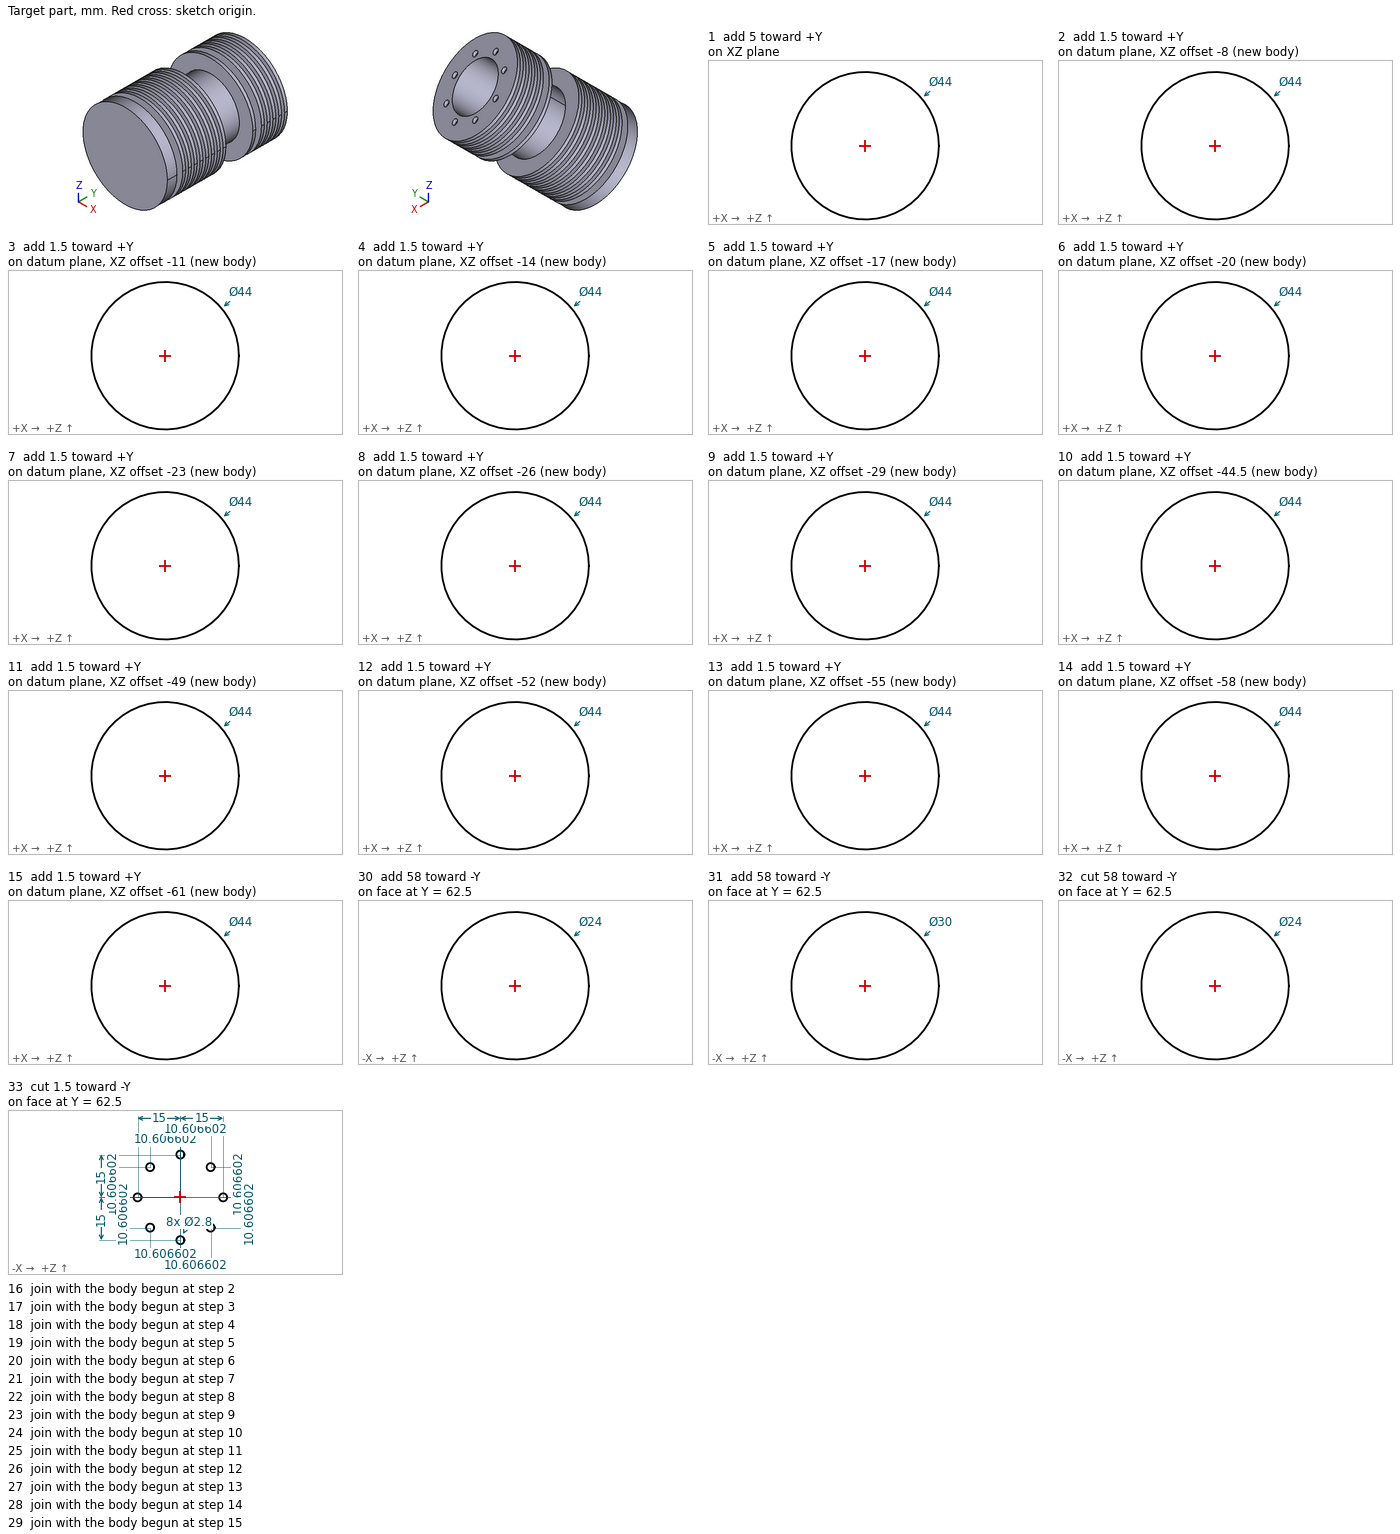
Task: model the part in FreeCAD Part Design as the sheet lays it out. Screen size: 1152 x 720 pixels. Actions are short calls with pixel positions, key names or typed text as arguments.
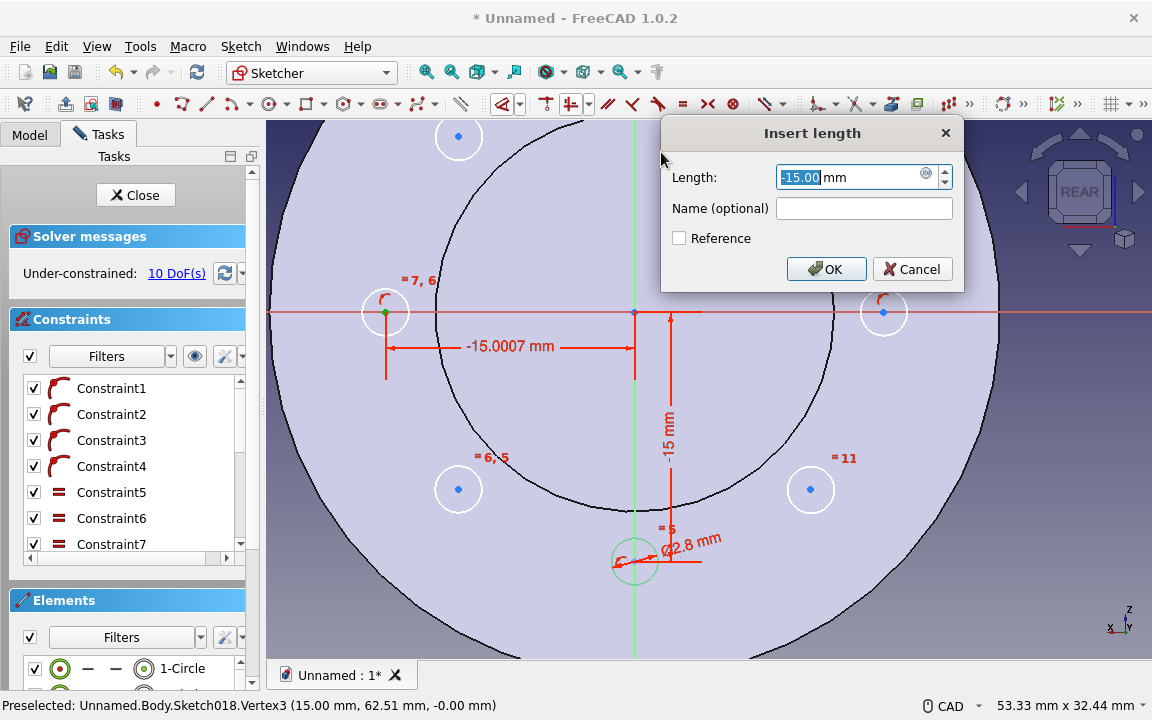
text(-15)
key(Return)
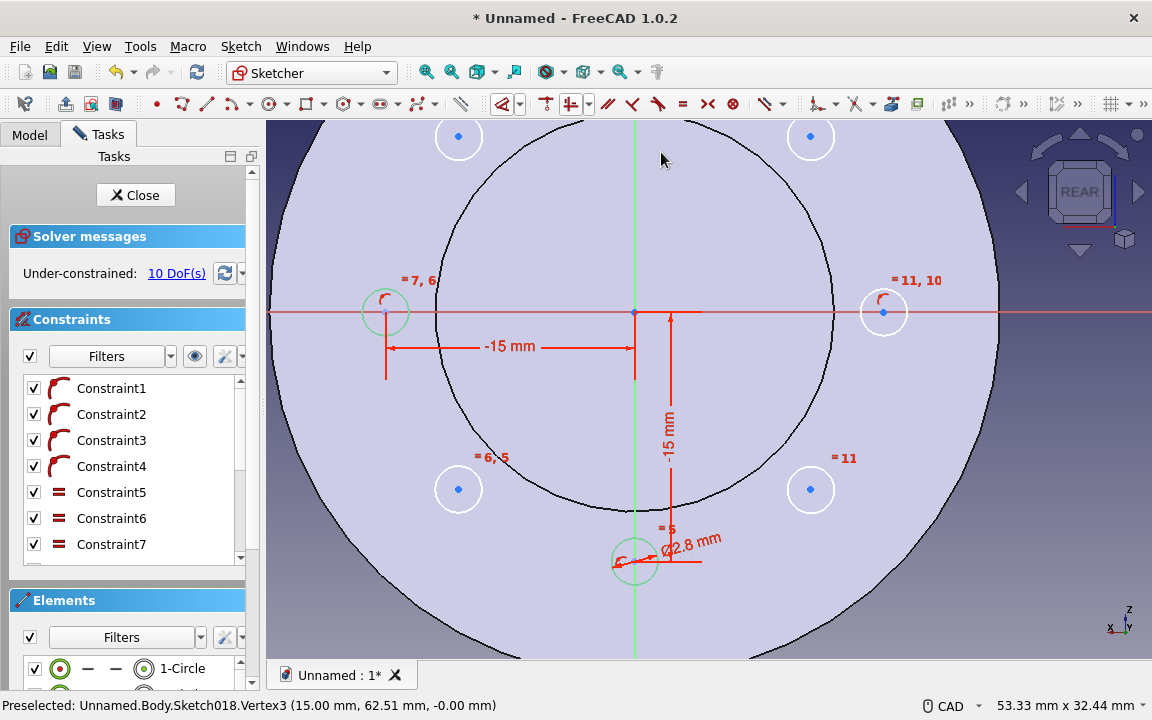
scroll(652, 546, down, 2)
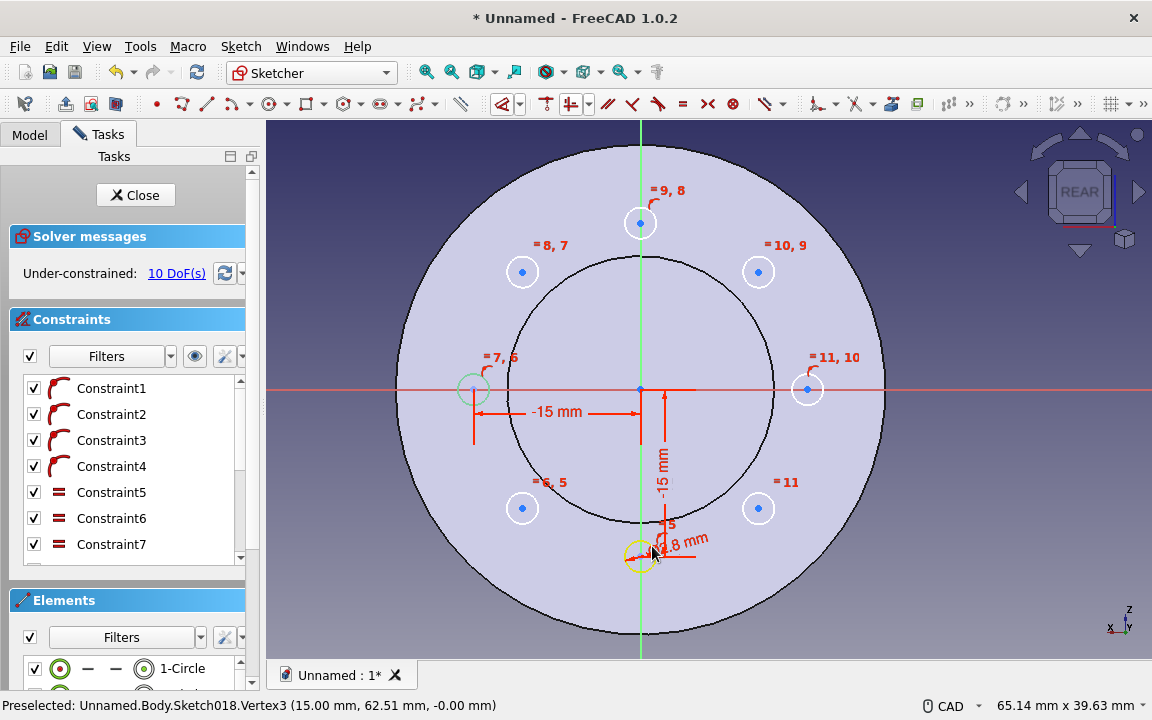
click(641, 223)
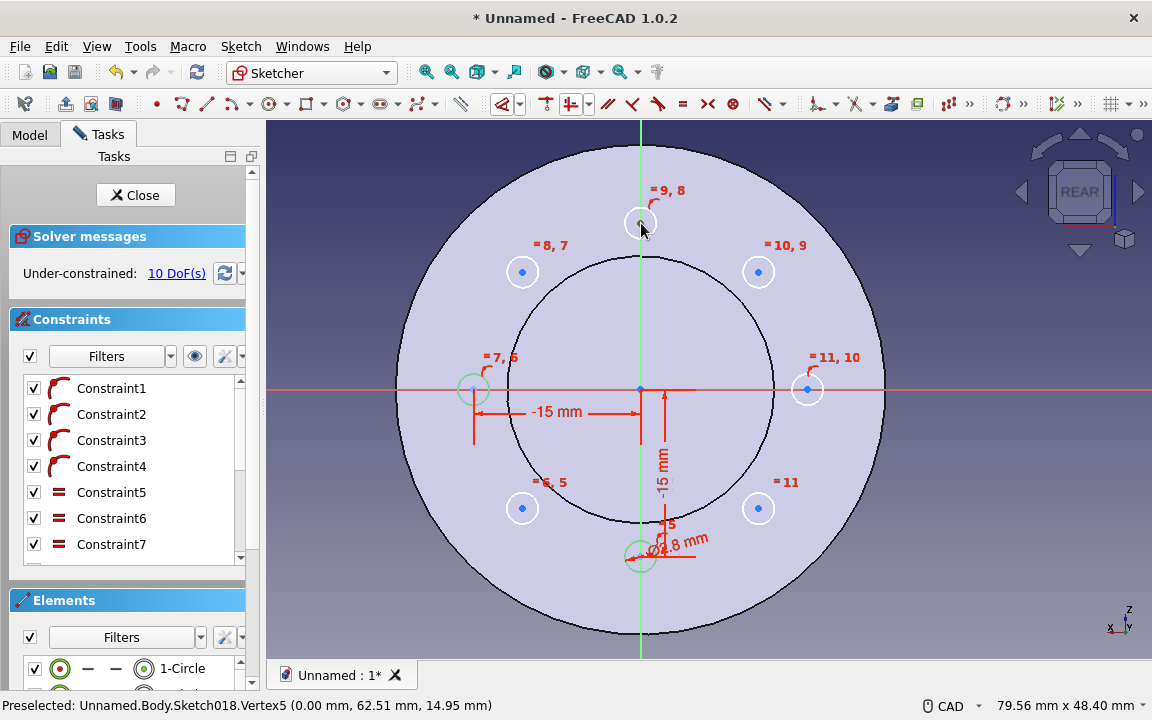
key(i)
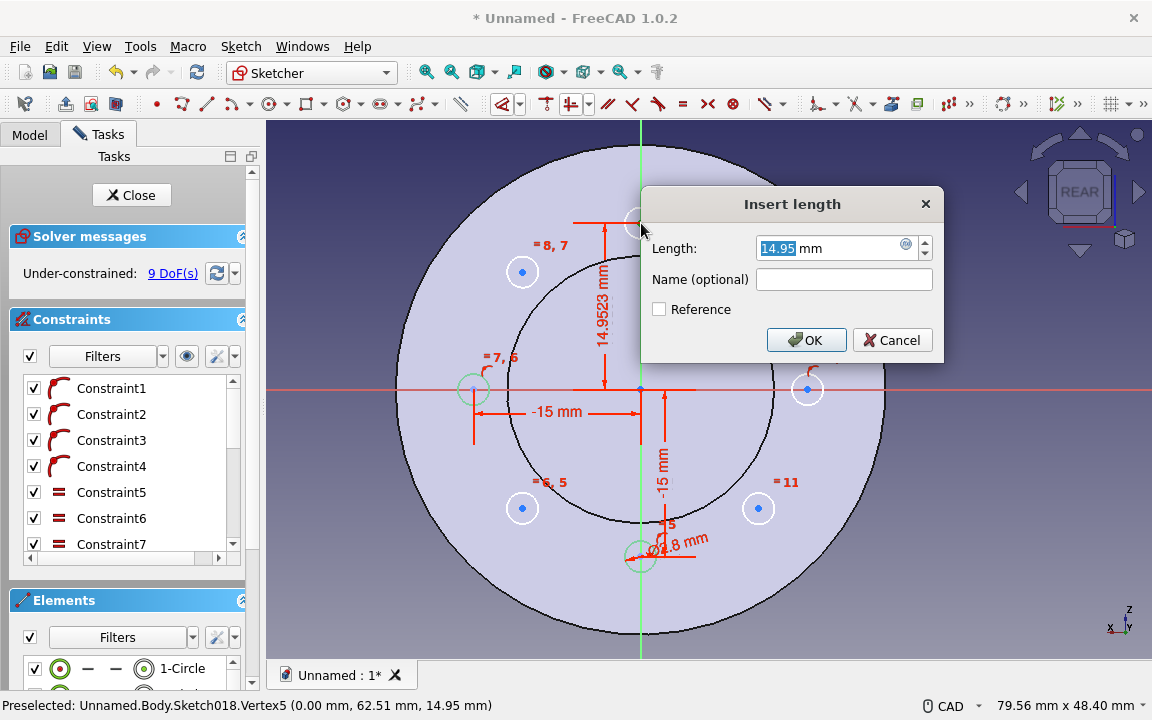
text(15)
key(Return)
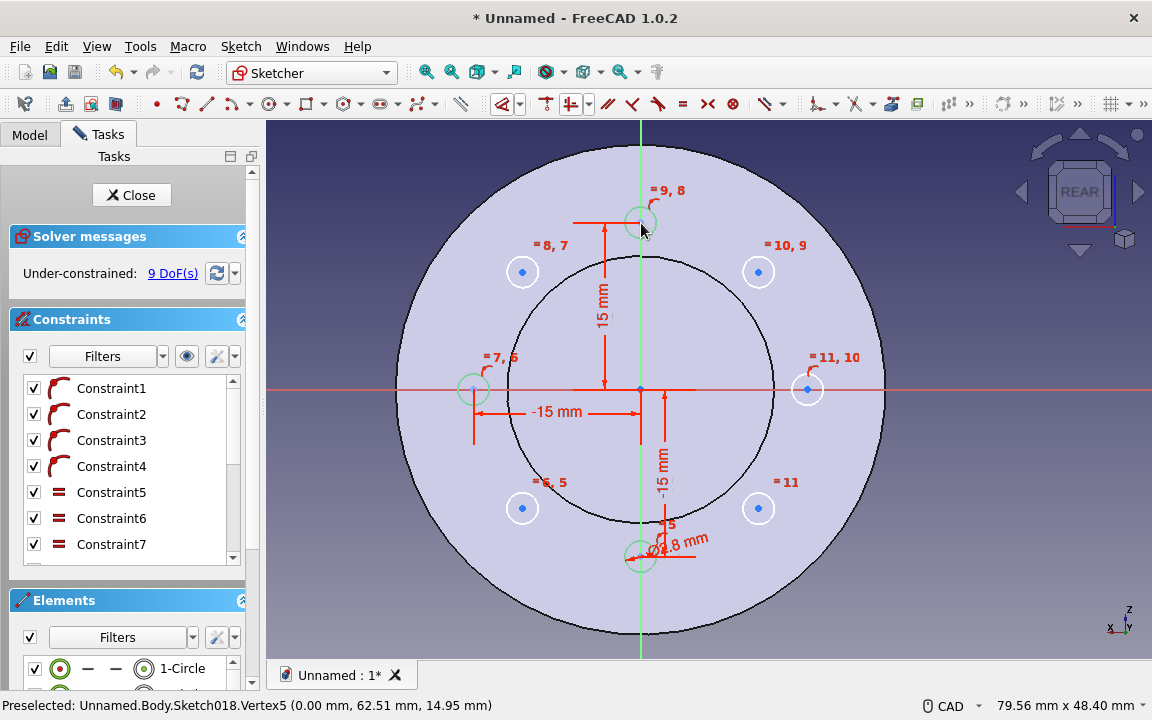
click(808, 390)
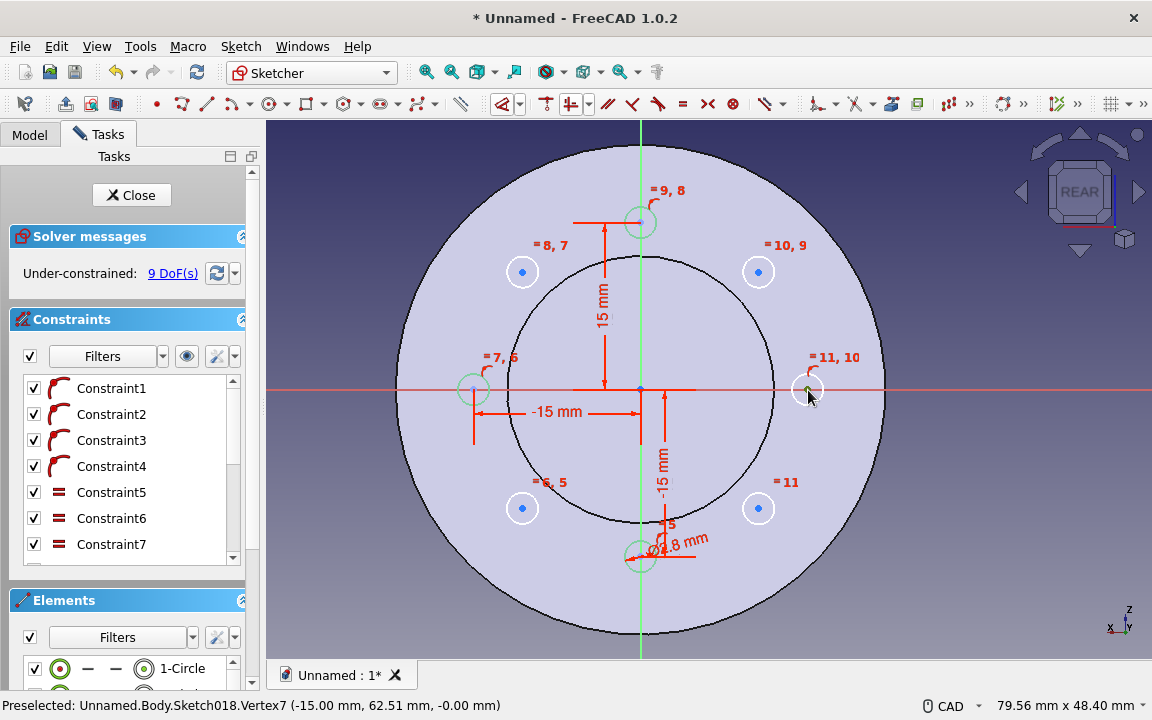
key(l)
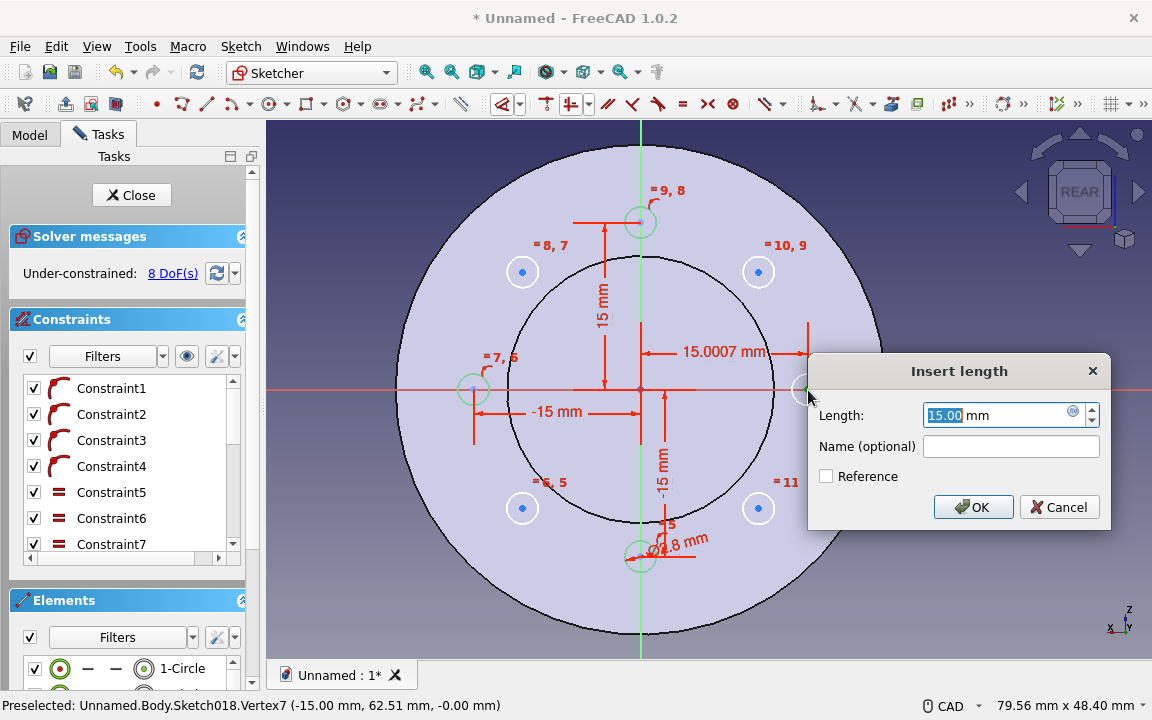
text(15)
key(Return)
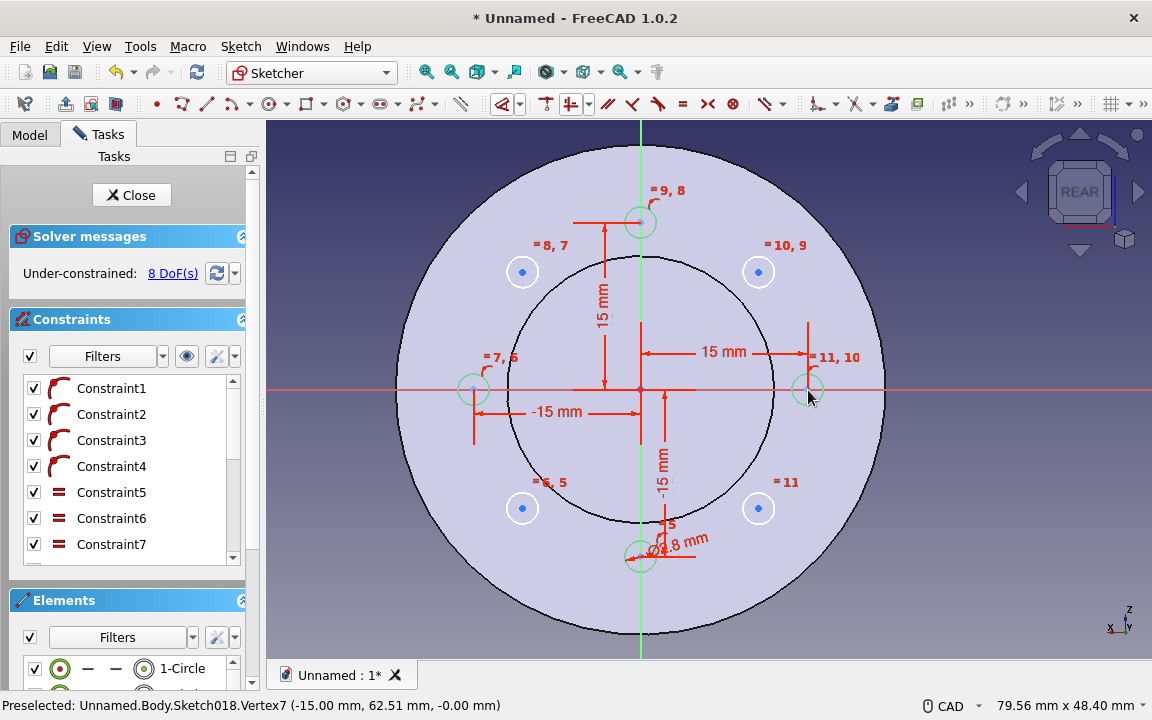
click(522, 508)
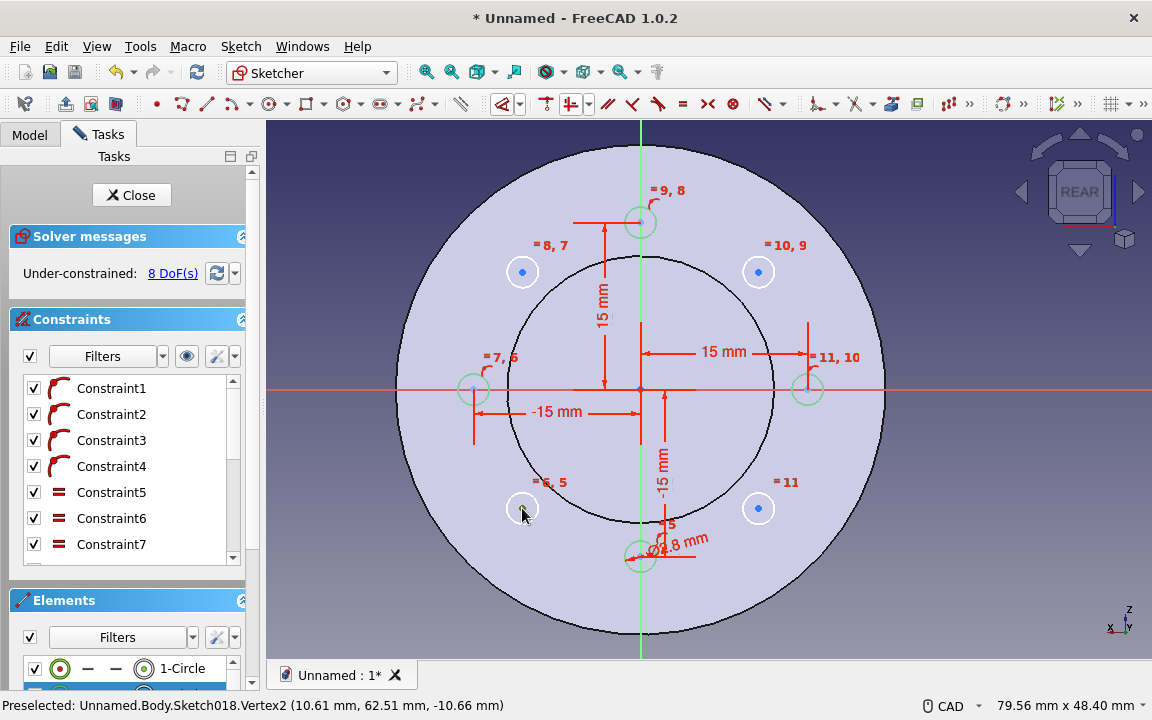
key(l)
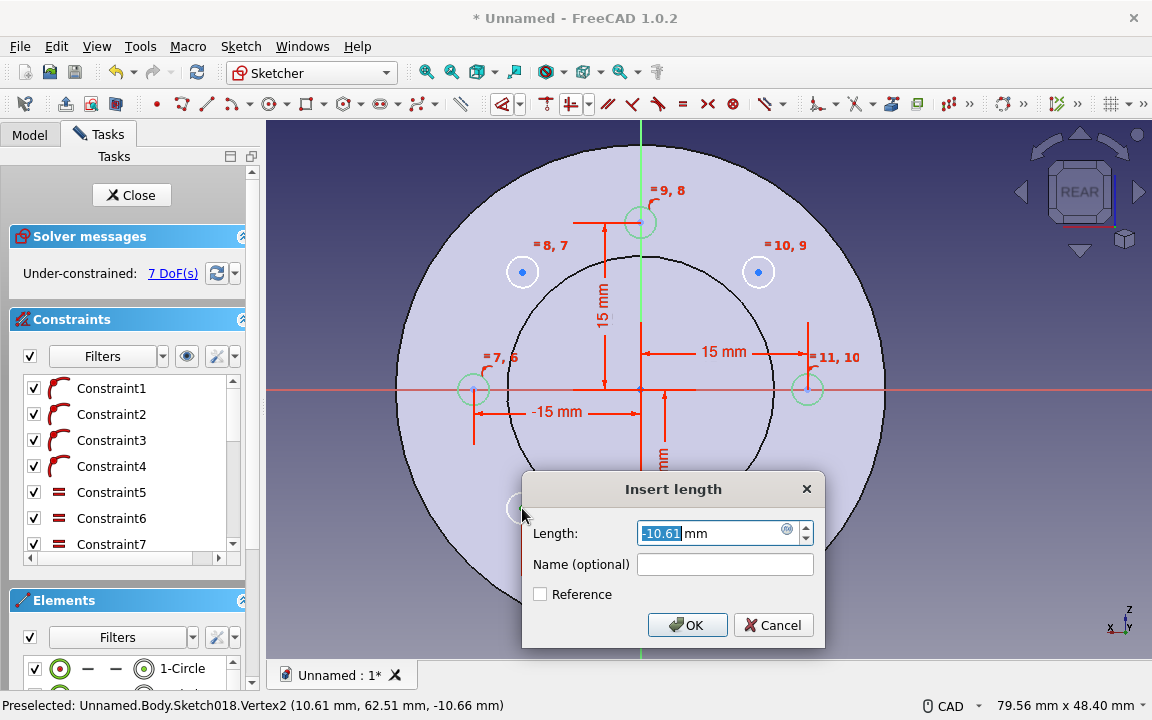
text(-10.606602)
key(Return)